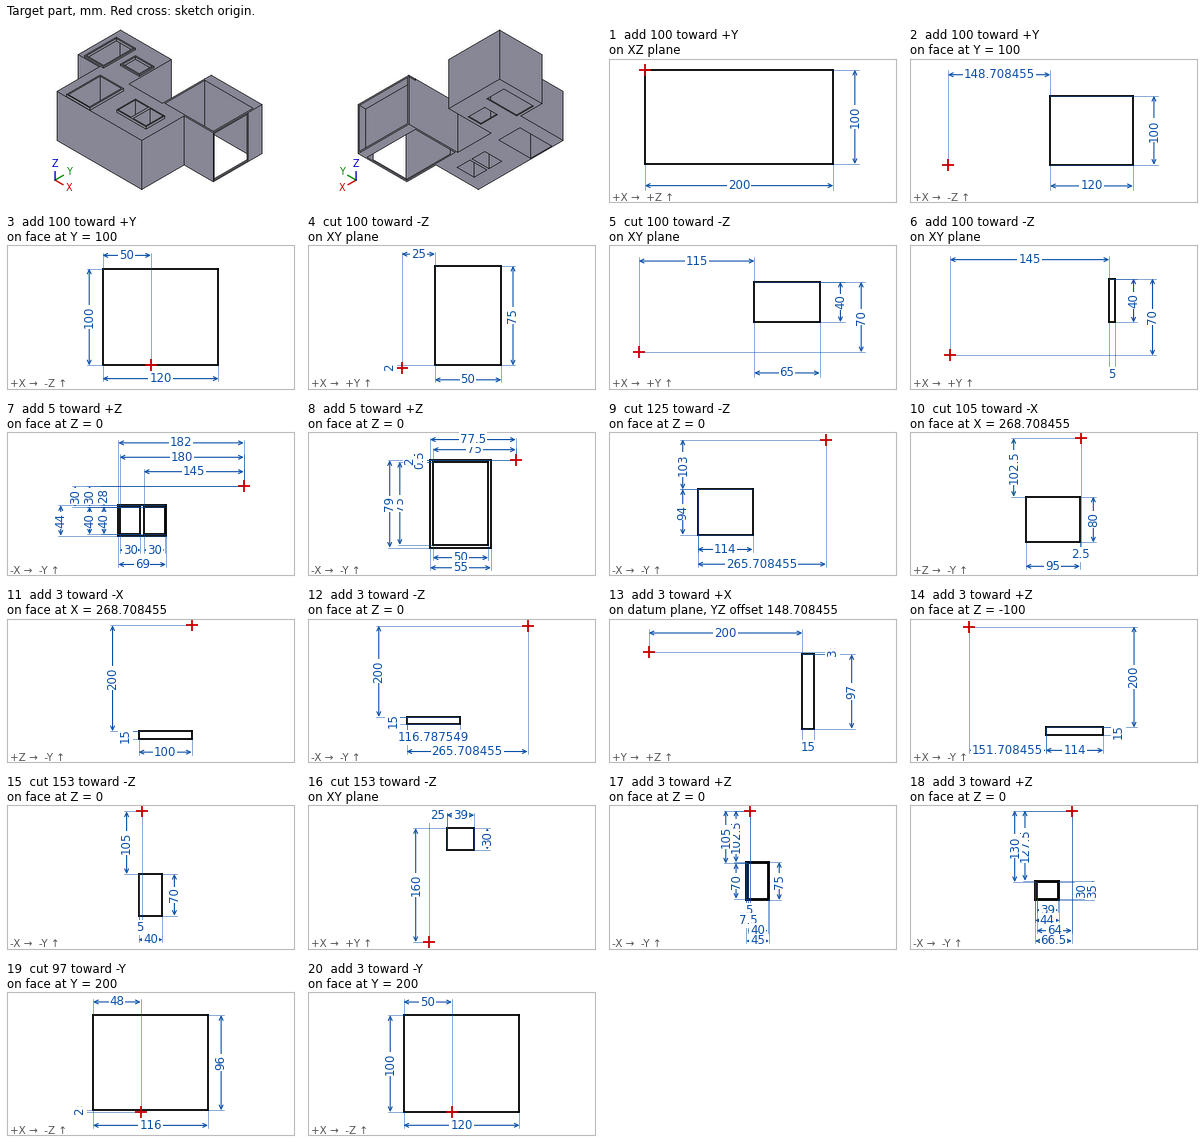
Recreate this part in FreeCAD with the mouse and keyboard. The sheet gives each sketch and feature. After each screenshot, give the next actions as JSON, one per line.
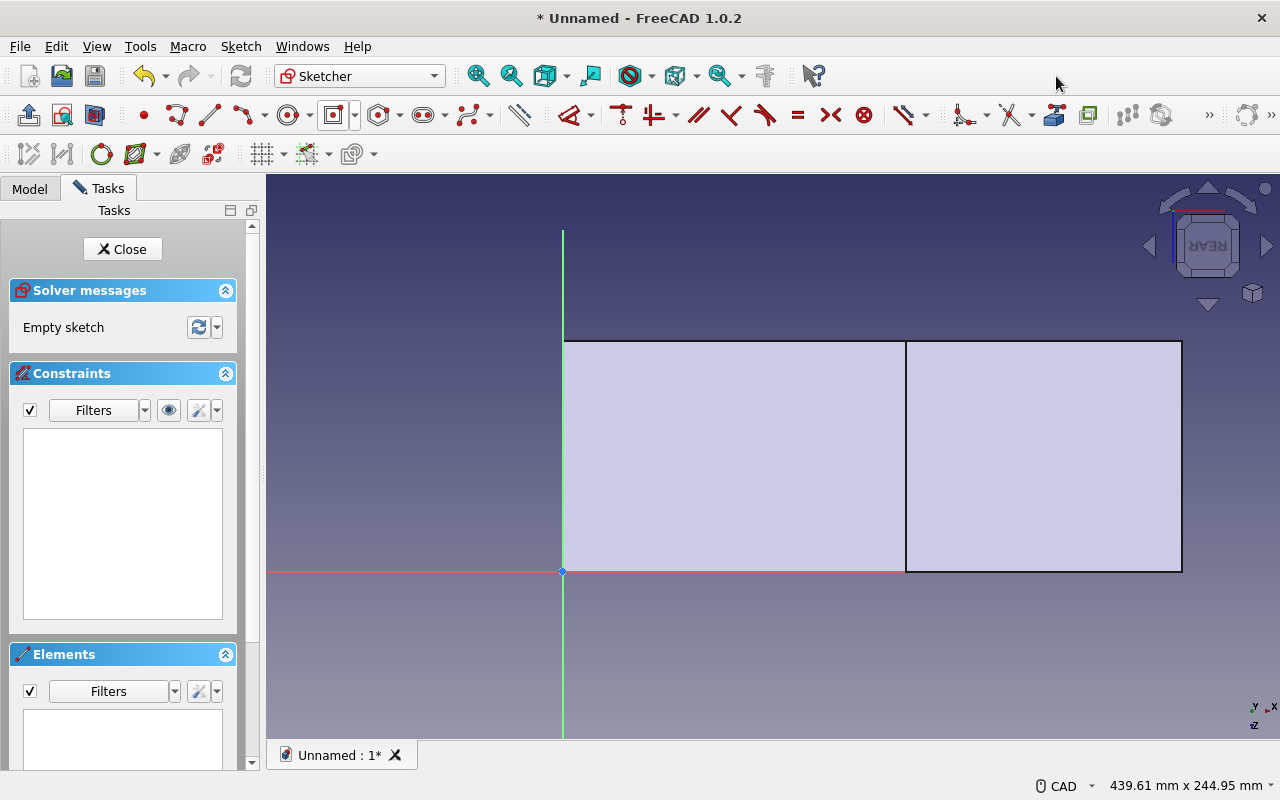
{"action": "scroll", "coordinate": [344, 456], "scroll_direction": "up", "scroll_amount": 2}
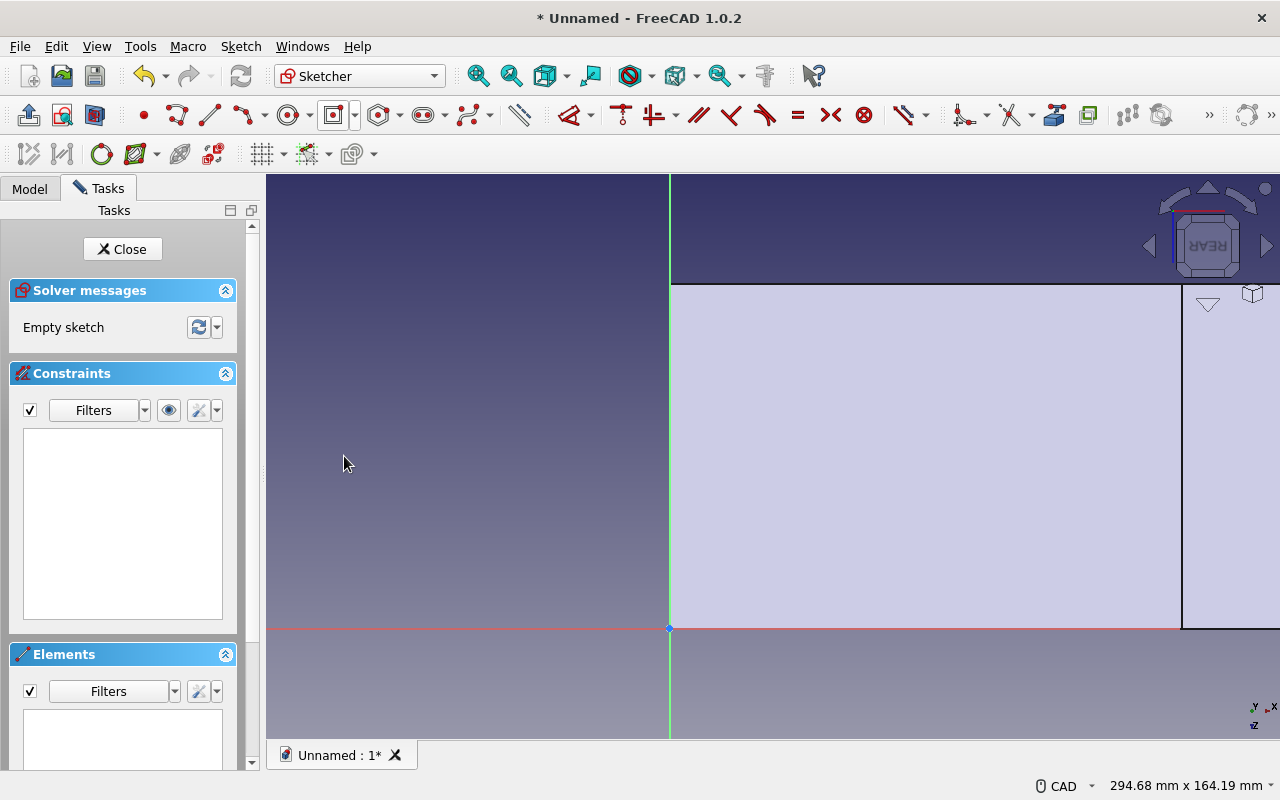
{"action": "left_click", "coordinate": [354, 116]}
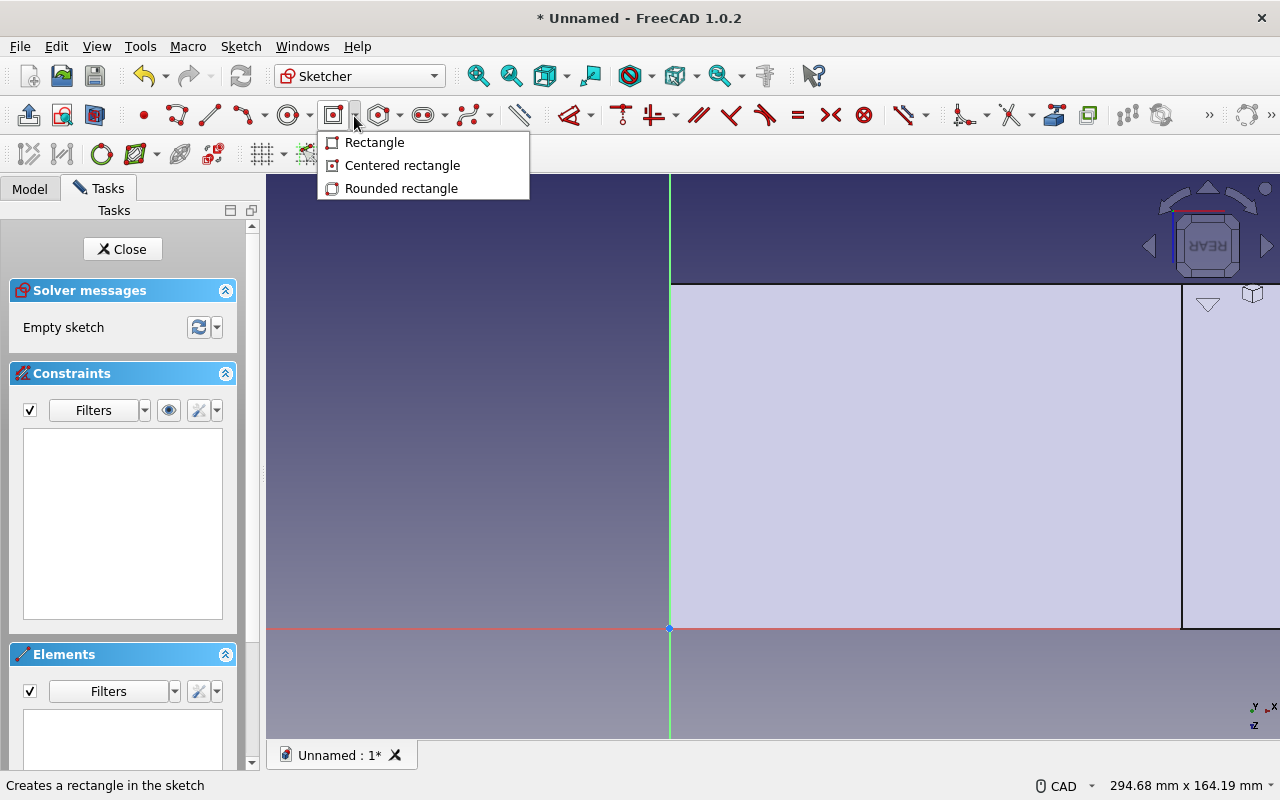
{"action": "left_click", "coordinate": [424, 142]}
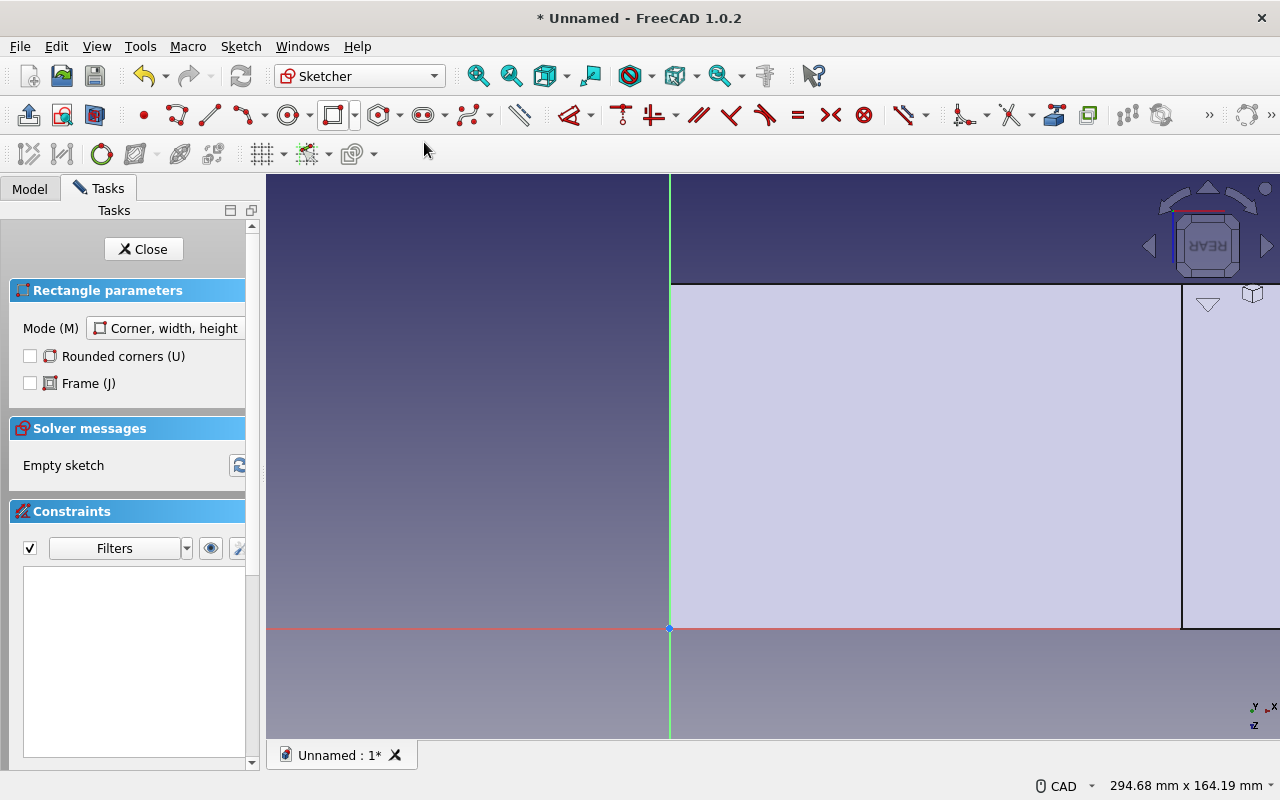
{"action": "left_click", "coordinate": [498, 284]}
{"action": "left_click", "coordinate": [911, 629]}
{"action": "key", "text": "Escape"}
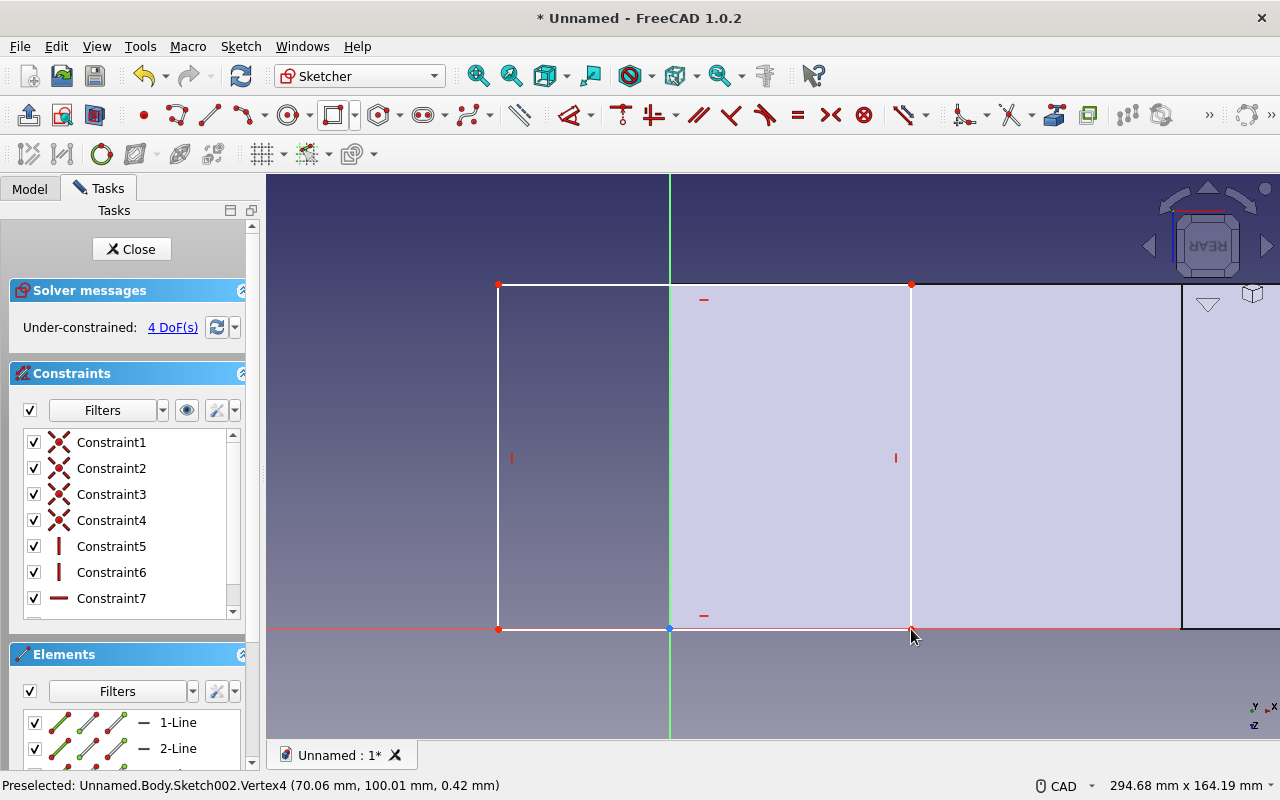
{"action": "left_click", "coordinate": [498, 630]}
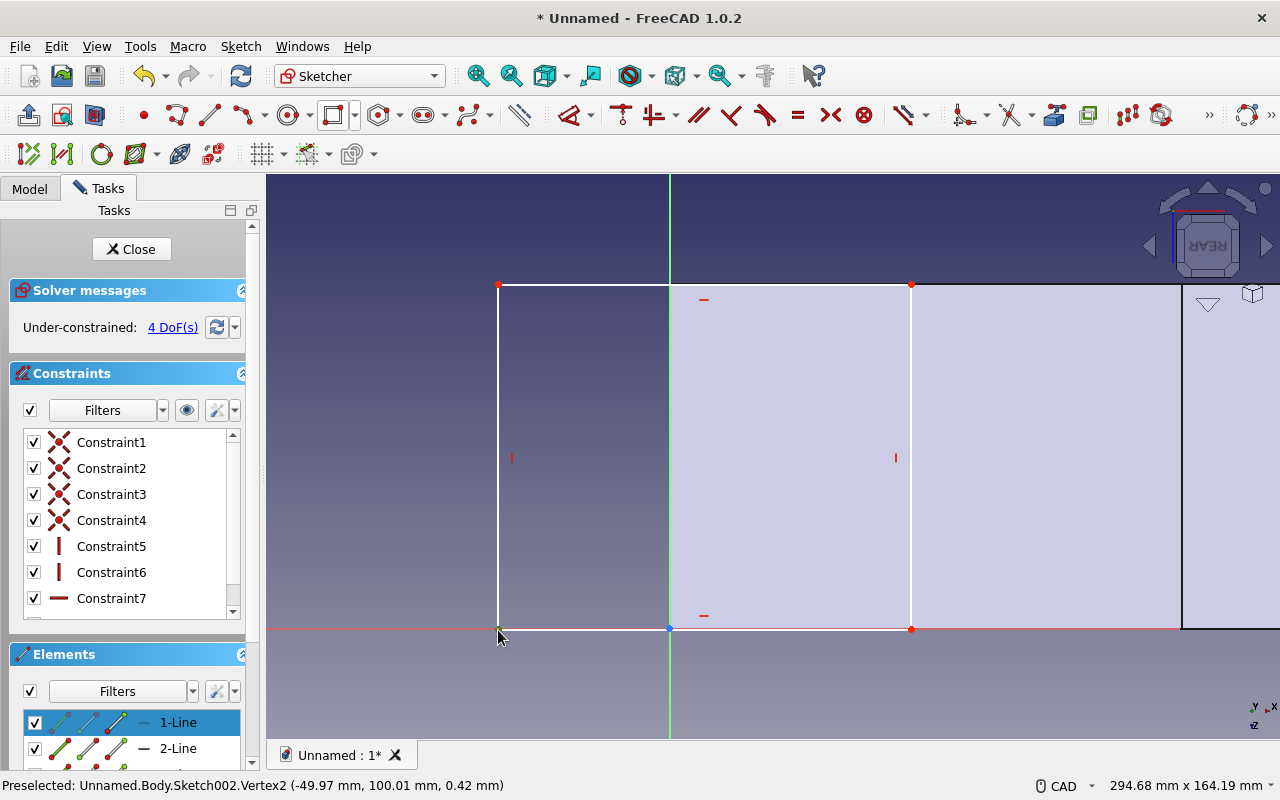
{"action": "left_click", "coordinate": [353, 629]}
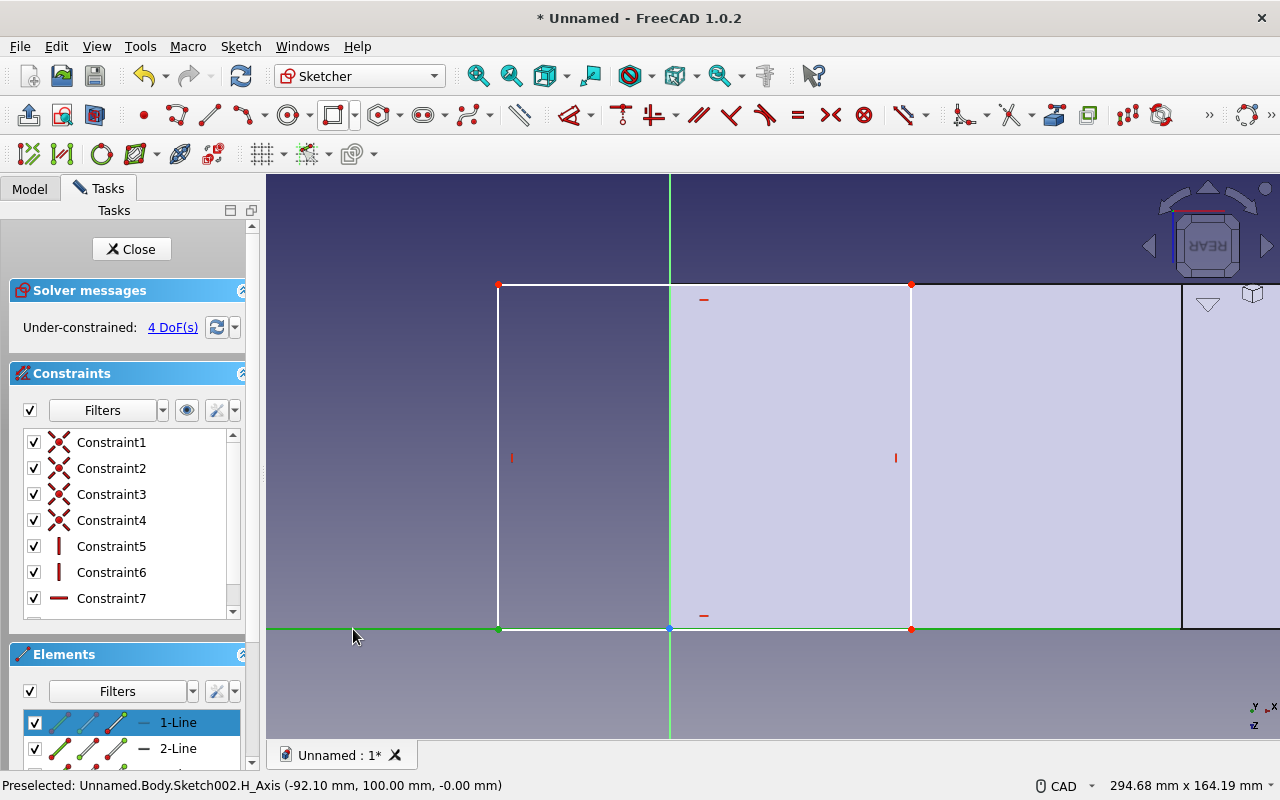
{"action": "left_click", "coordinate": [621, 116]}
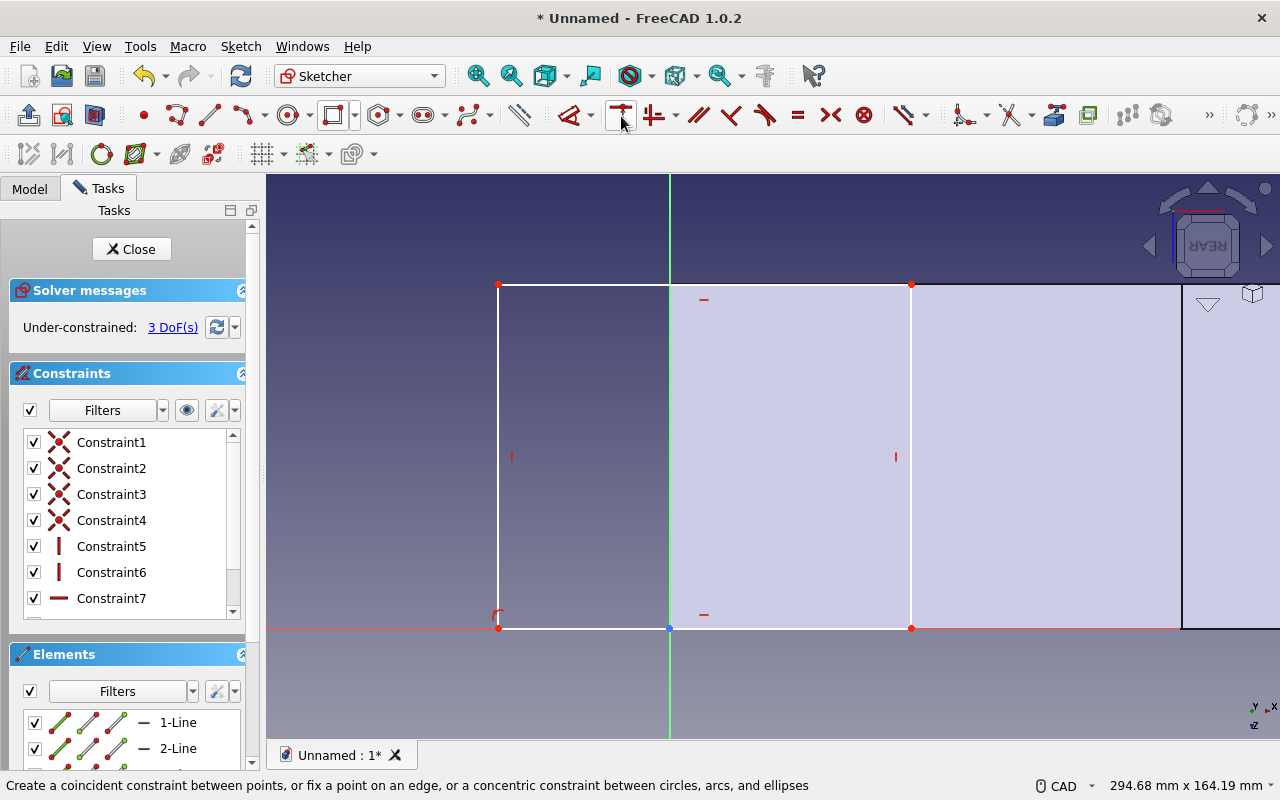
{"action": "left_click", "coordinate": [568, 116]}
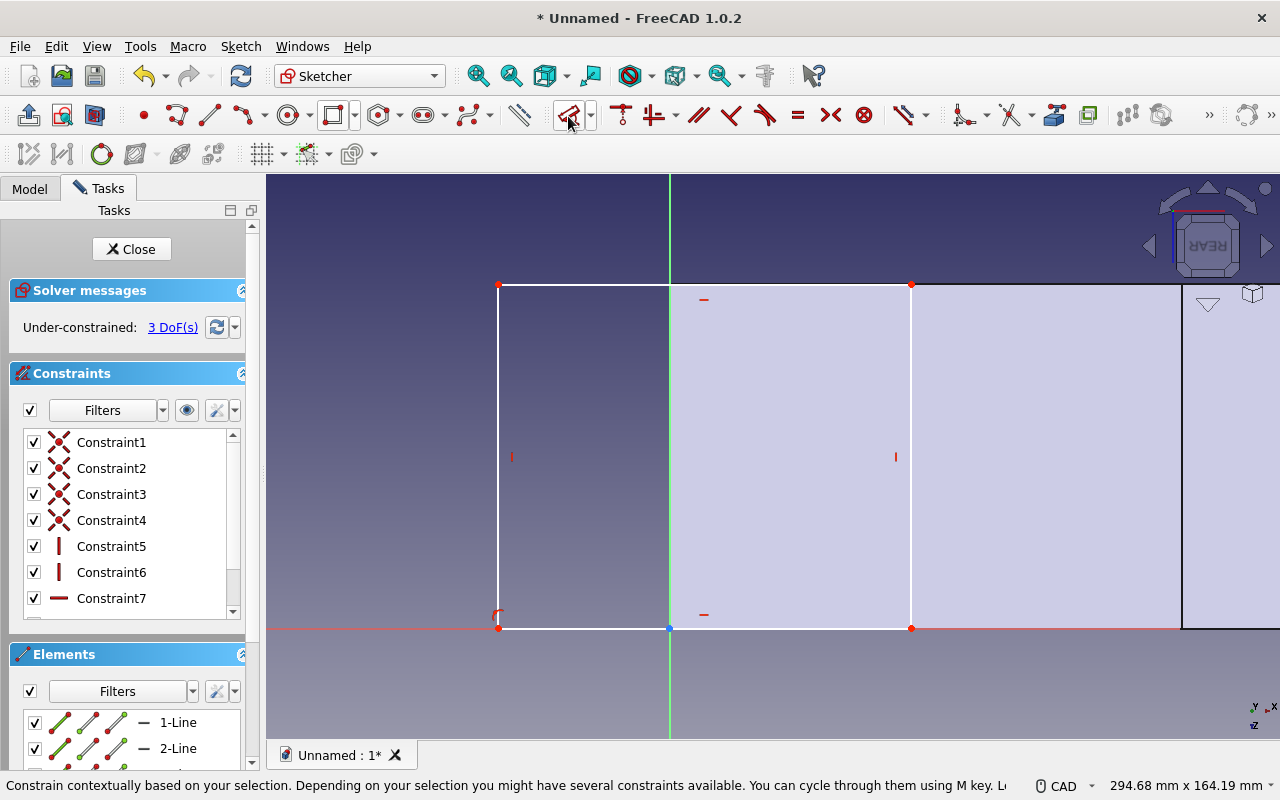
{"action": "left_click", "coordinate": [498, 388]}
{"action": "left_click", "coordinate": [464, 457]}